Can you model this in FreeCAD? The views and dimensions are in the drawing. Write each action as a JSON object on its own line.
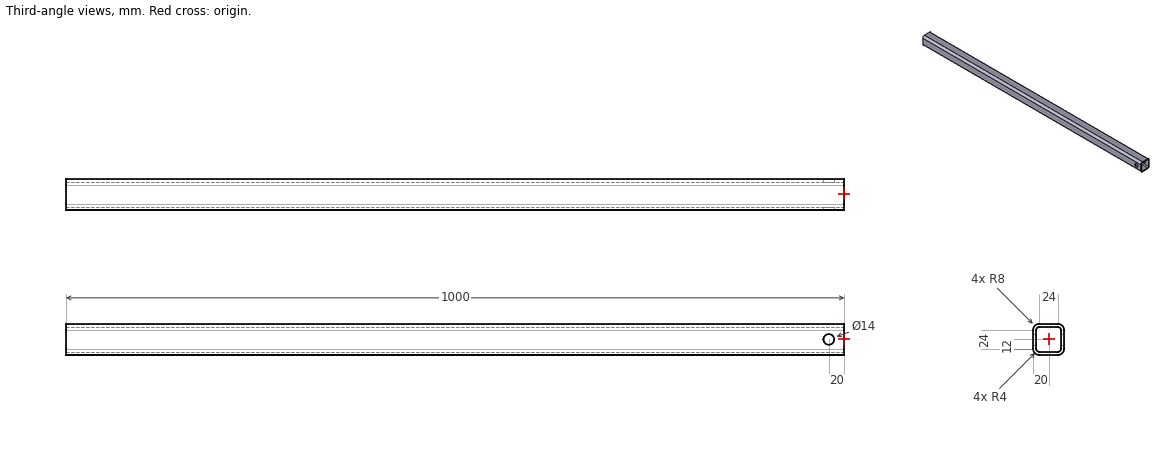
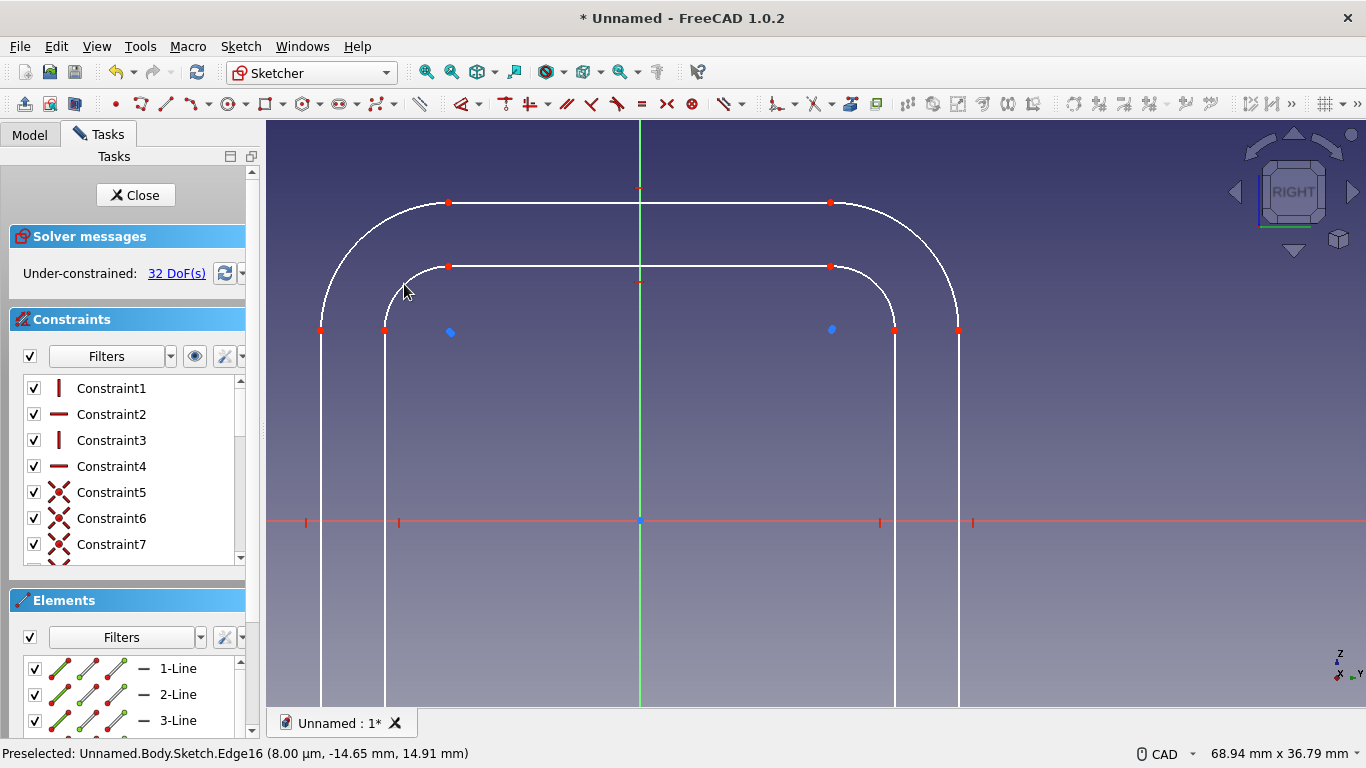
{"action": "left_click", "coordinate": [321, 599]}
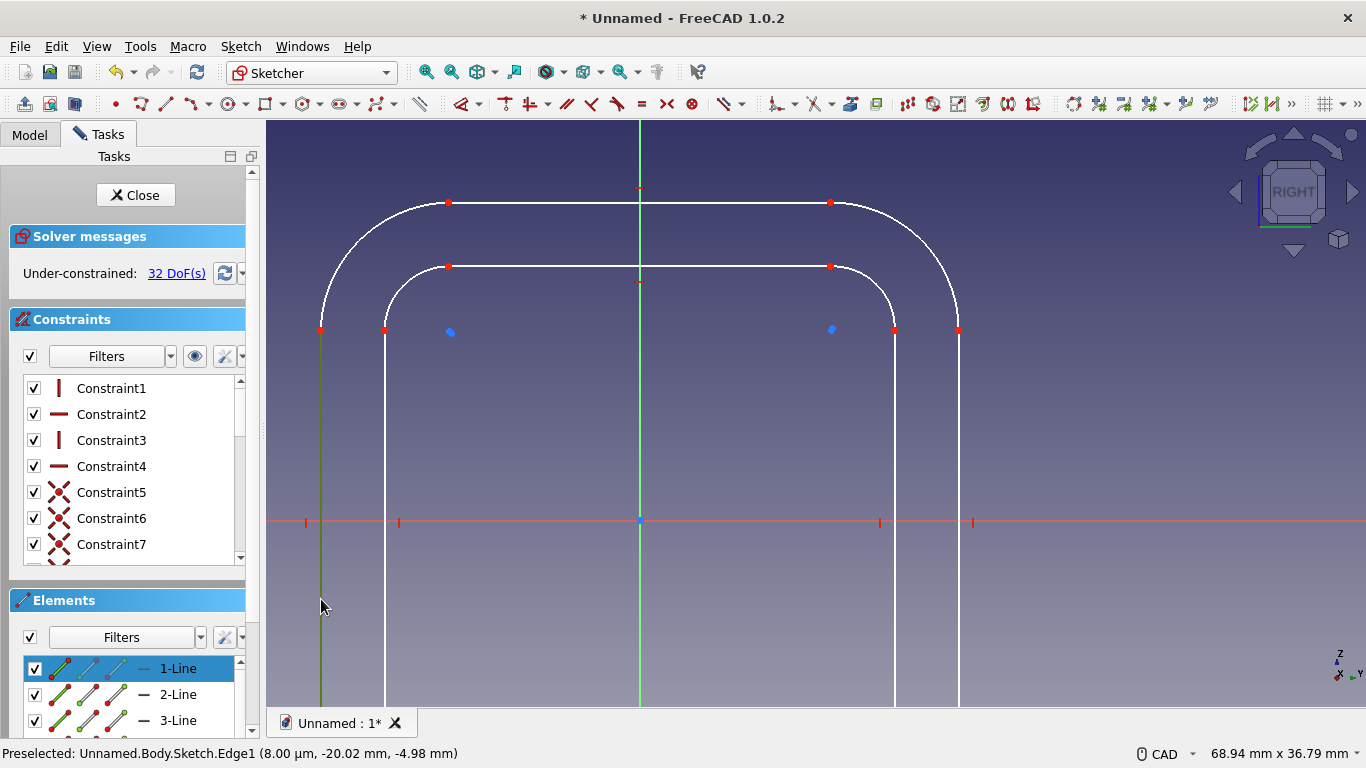
{"action": "left_click", "coordinate": [391, 217]}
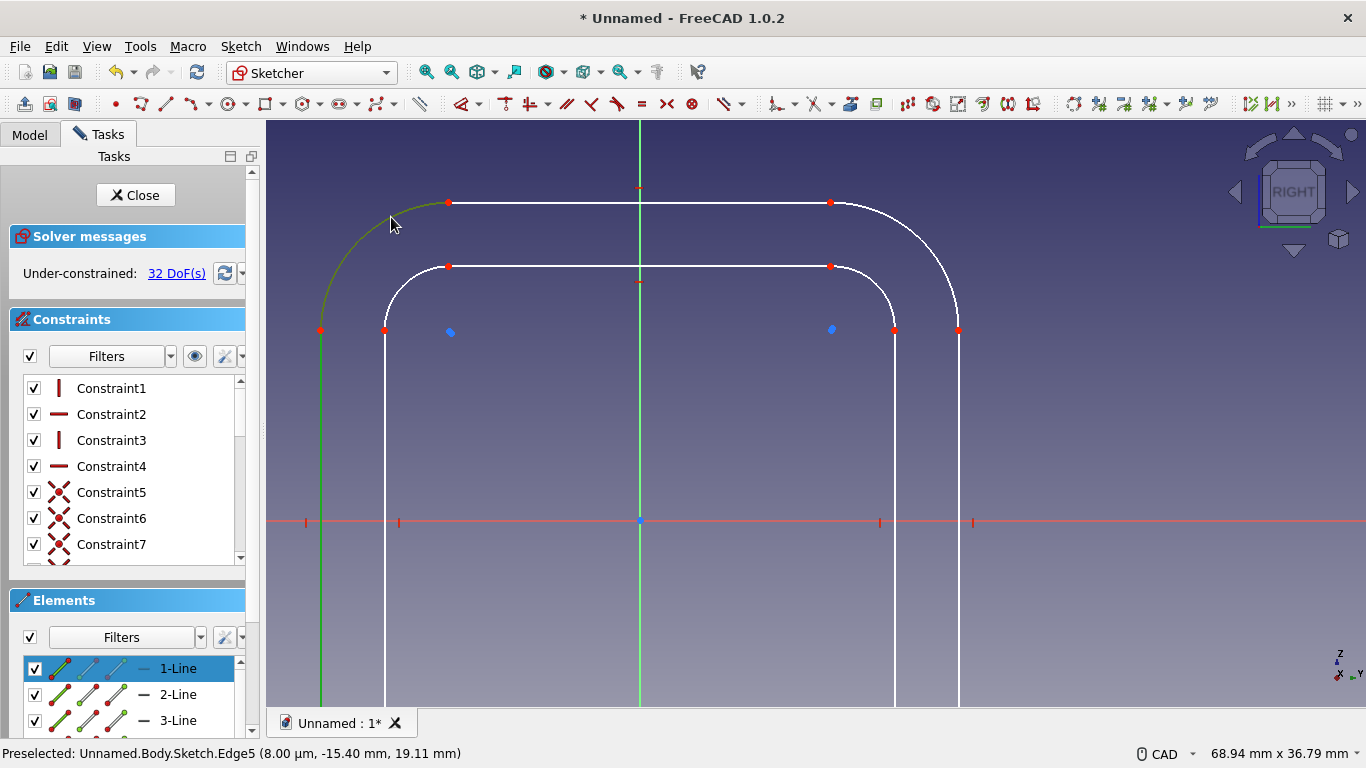
{"action": "left_click", "coordinate": [617, 104]}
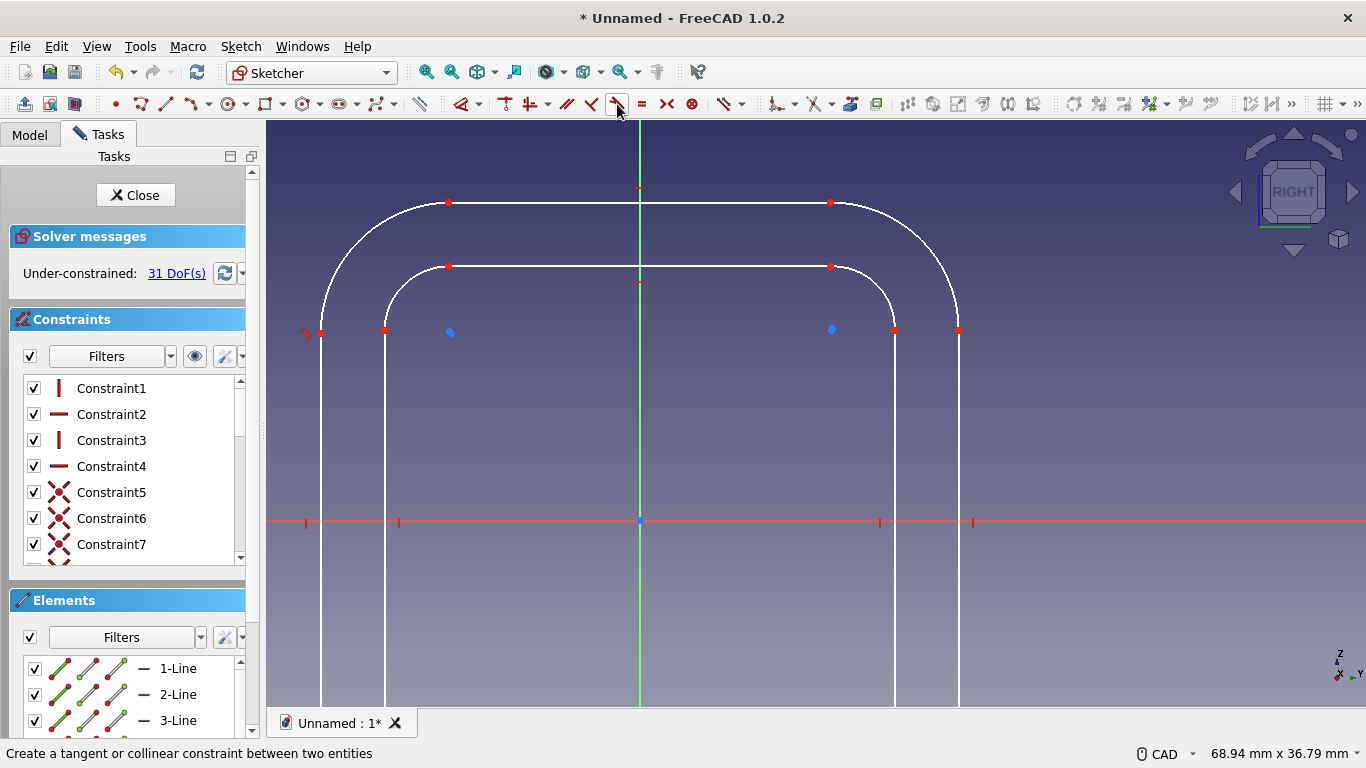
{"action": "left_click", "coordinate": [321, 600]}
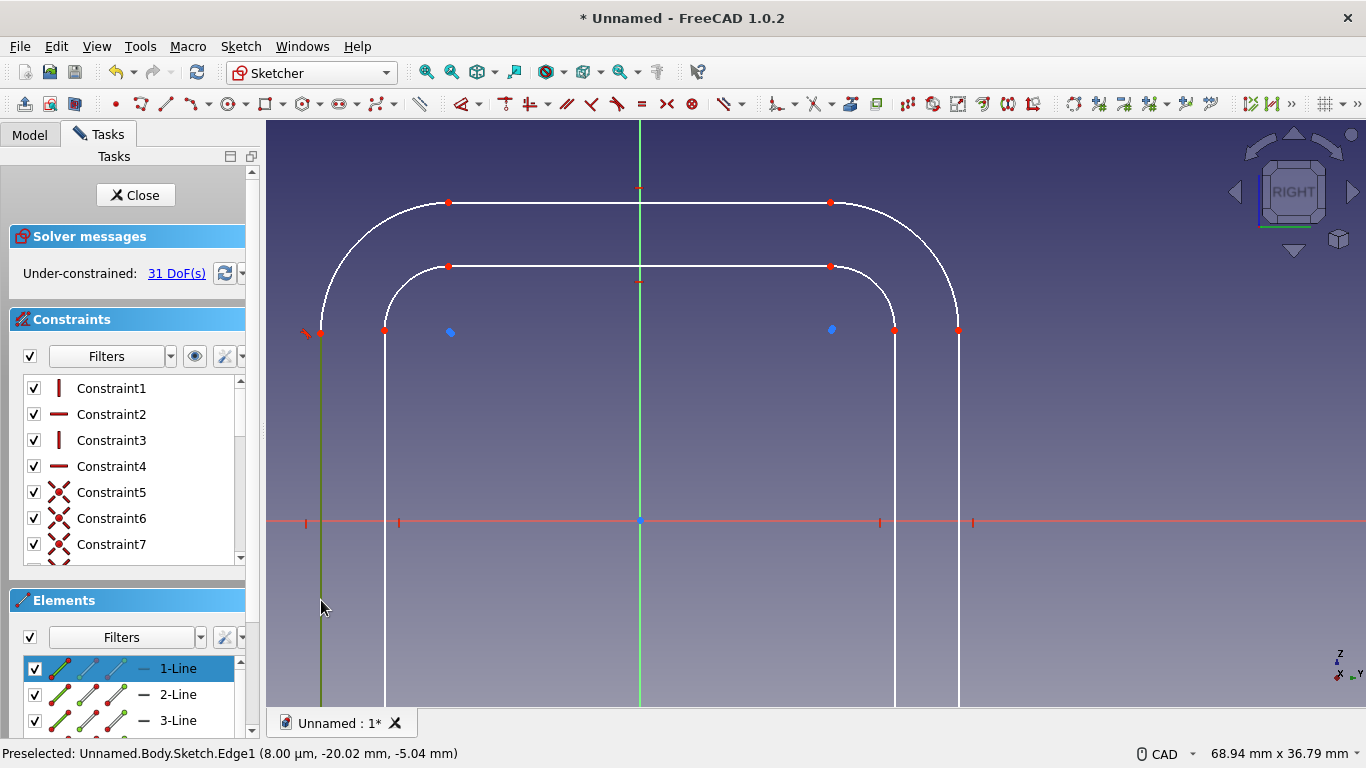
{"action": "scroll", "coordinate": [878, 283], "scroll_direction": "down", "scroll_amount": 3}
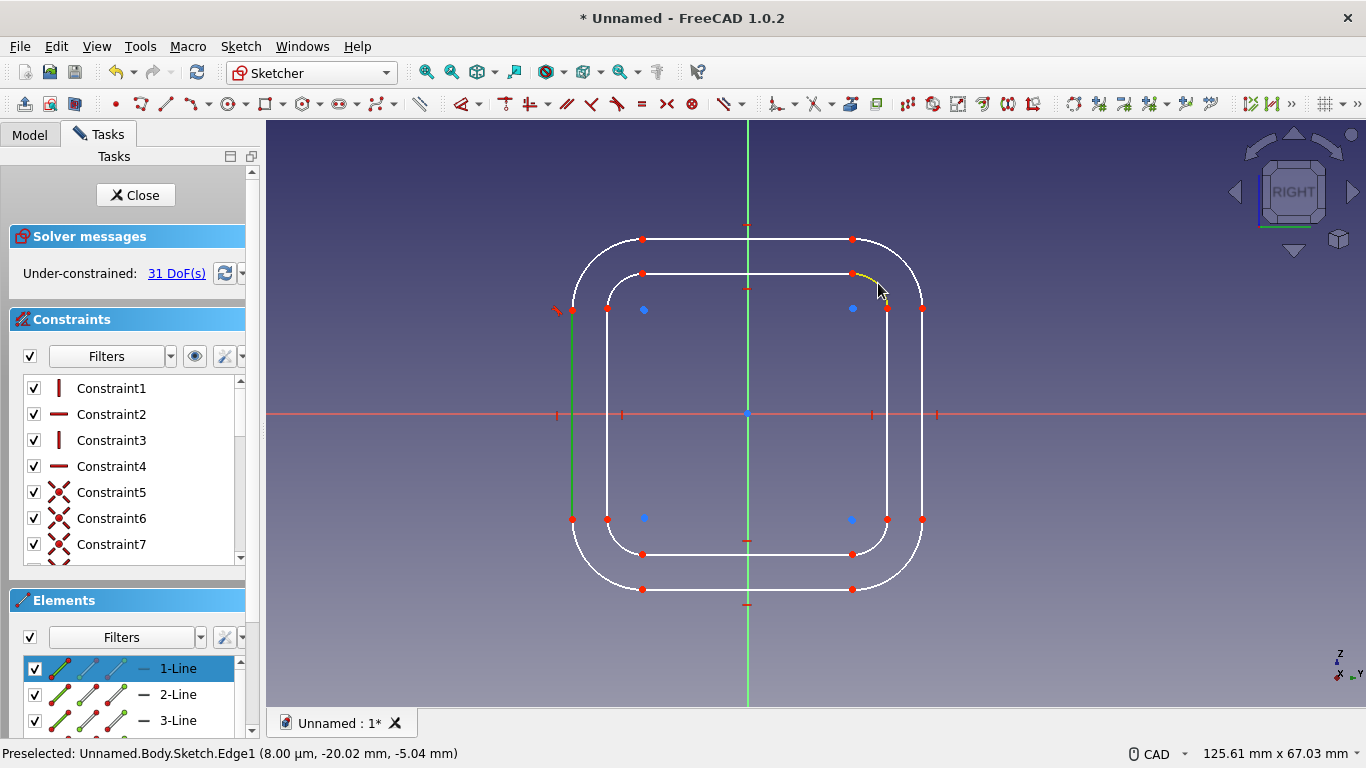
{"action": "left_click", "coordinate": [581, 551]}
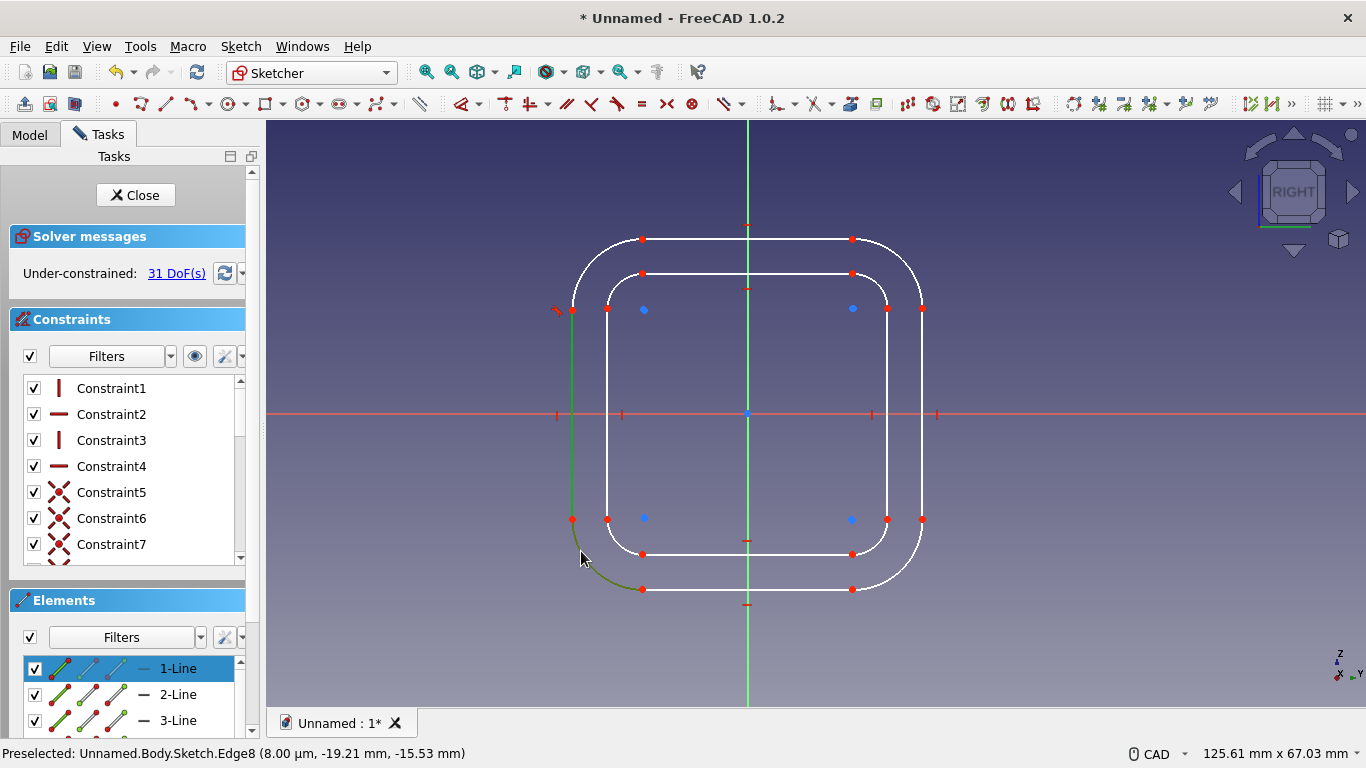
{"action": "left_click", "coordinate": [617, 104]}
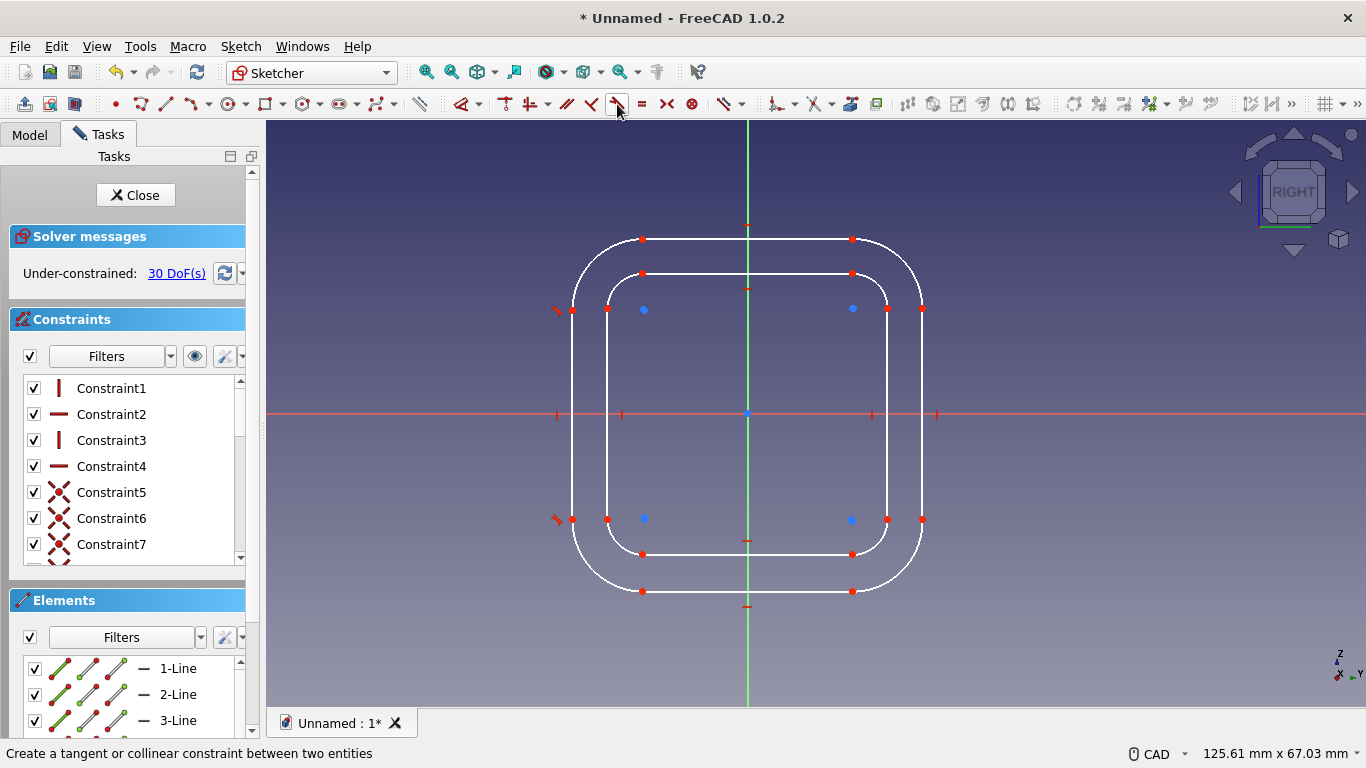
{"action": "left_click", "coordinate": [705, 239]}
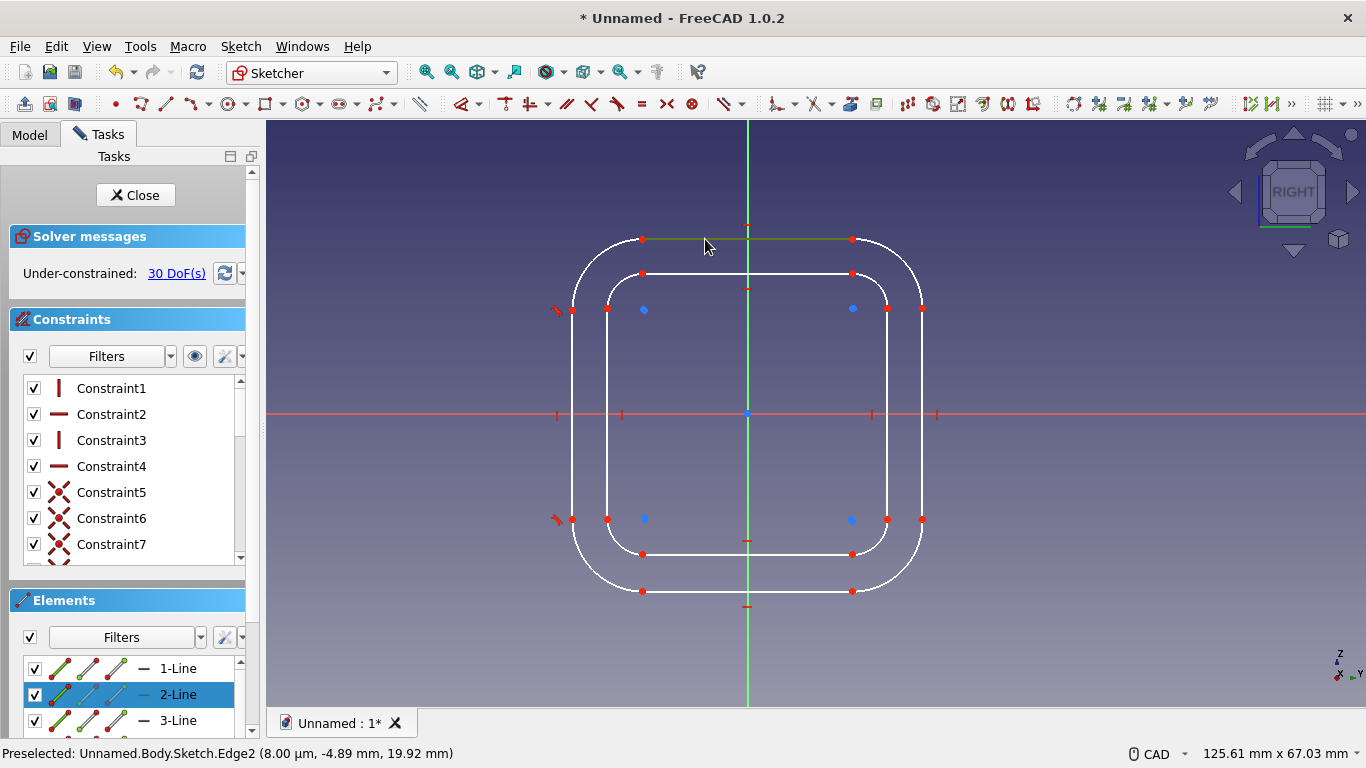
{"action": "left_click", "coordinate": [611, 247]}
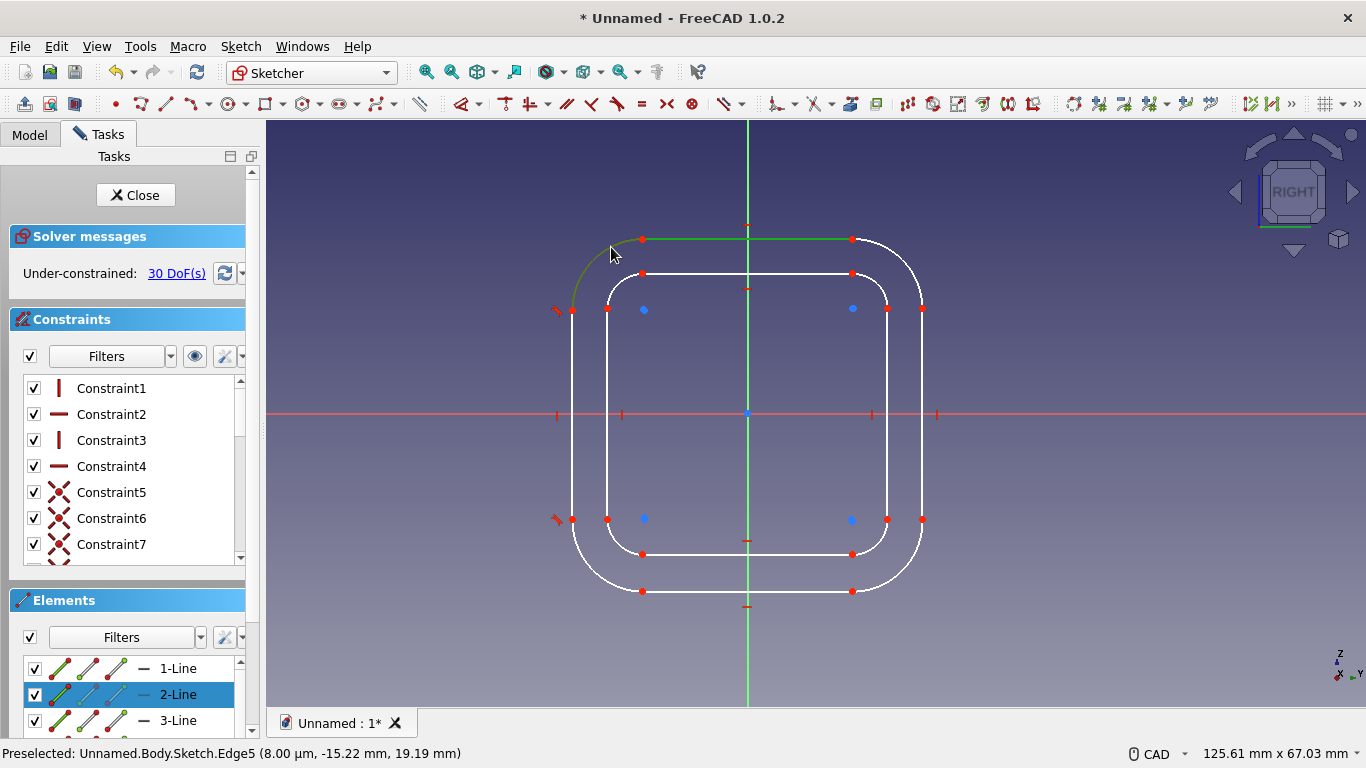
{"action": "left_click", "coordinate": [617, 104]}